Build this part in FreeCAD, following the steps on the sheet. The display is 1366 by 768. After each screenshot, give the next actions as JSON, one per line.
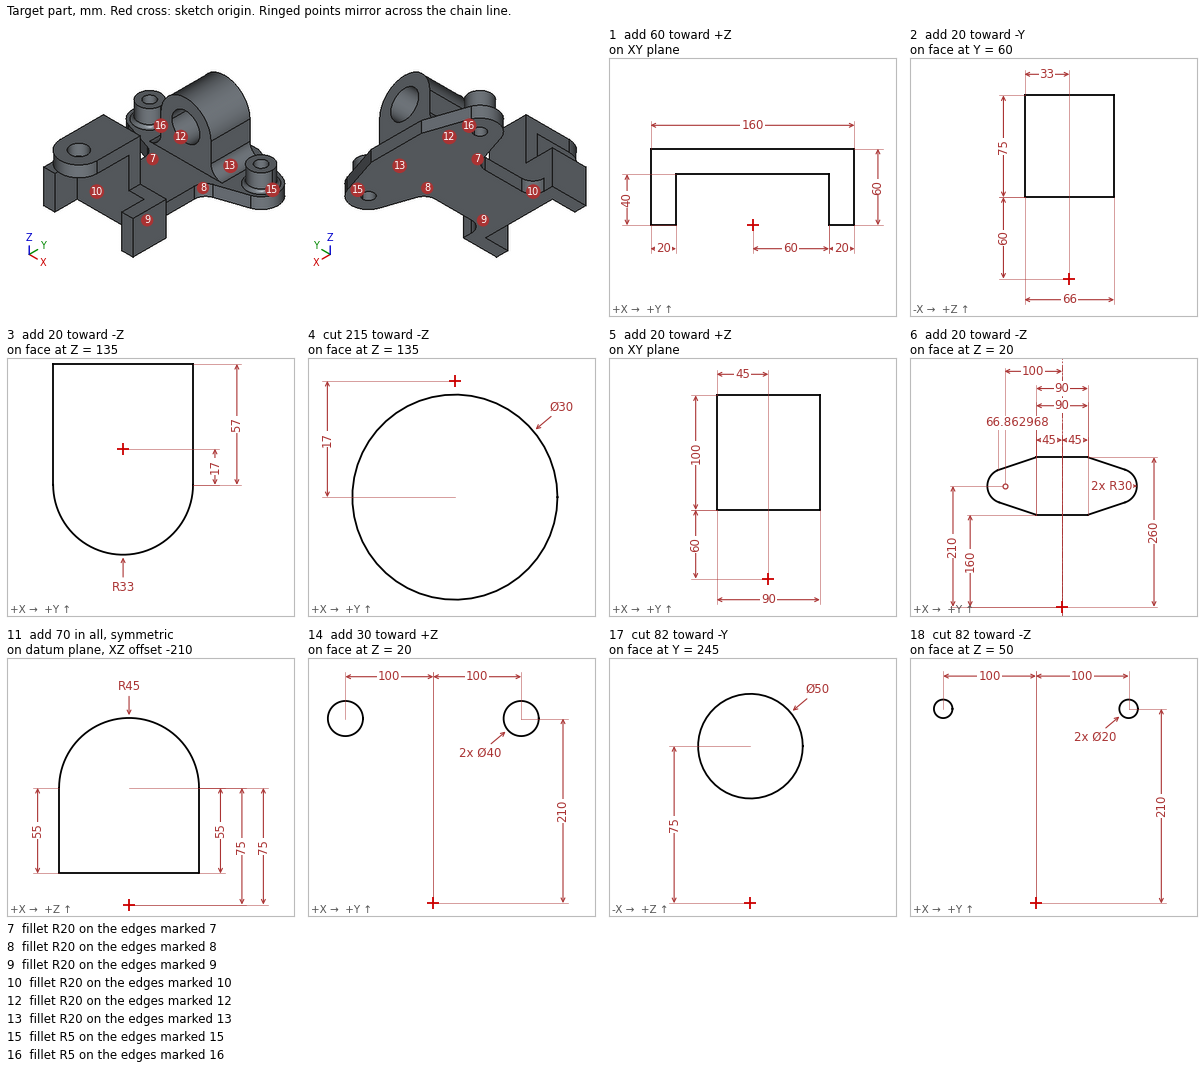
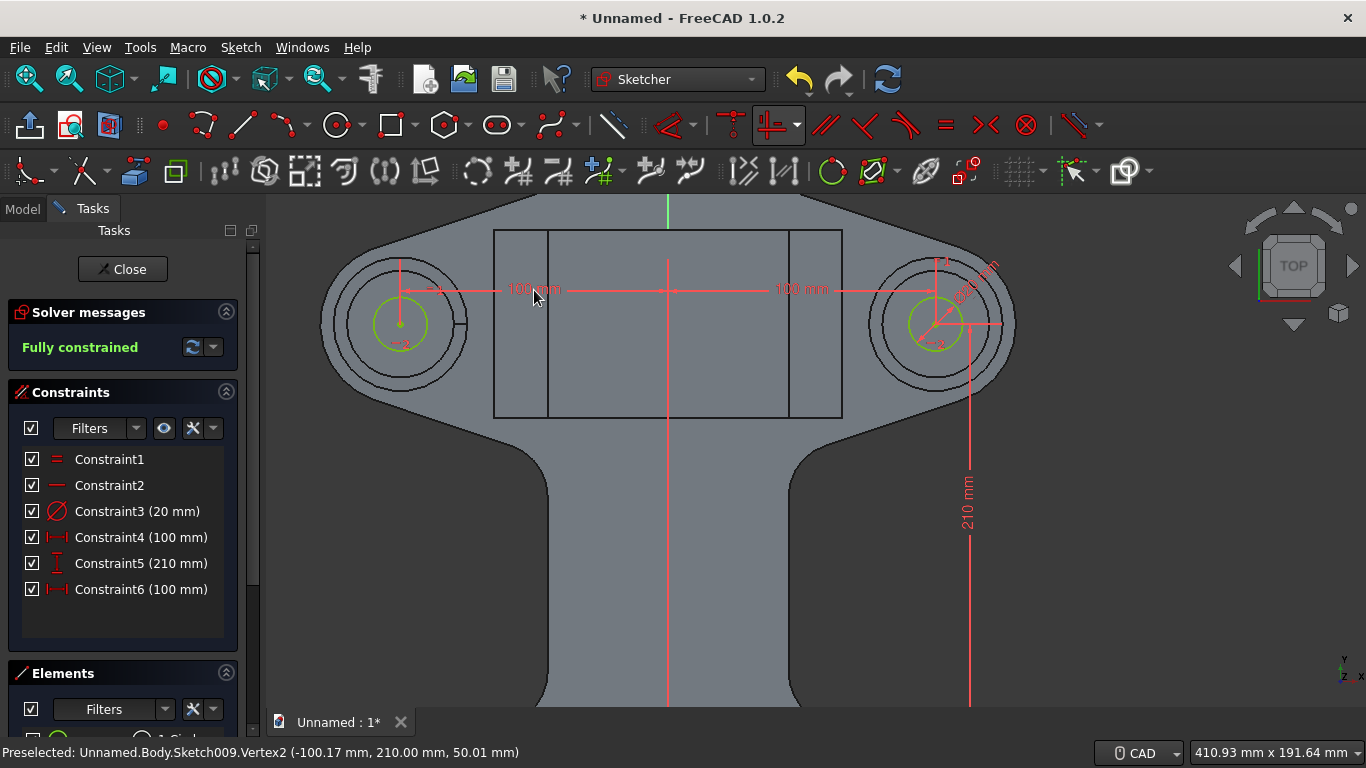
{"action": "left_click", "coordinate": [123, 269]}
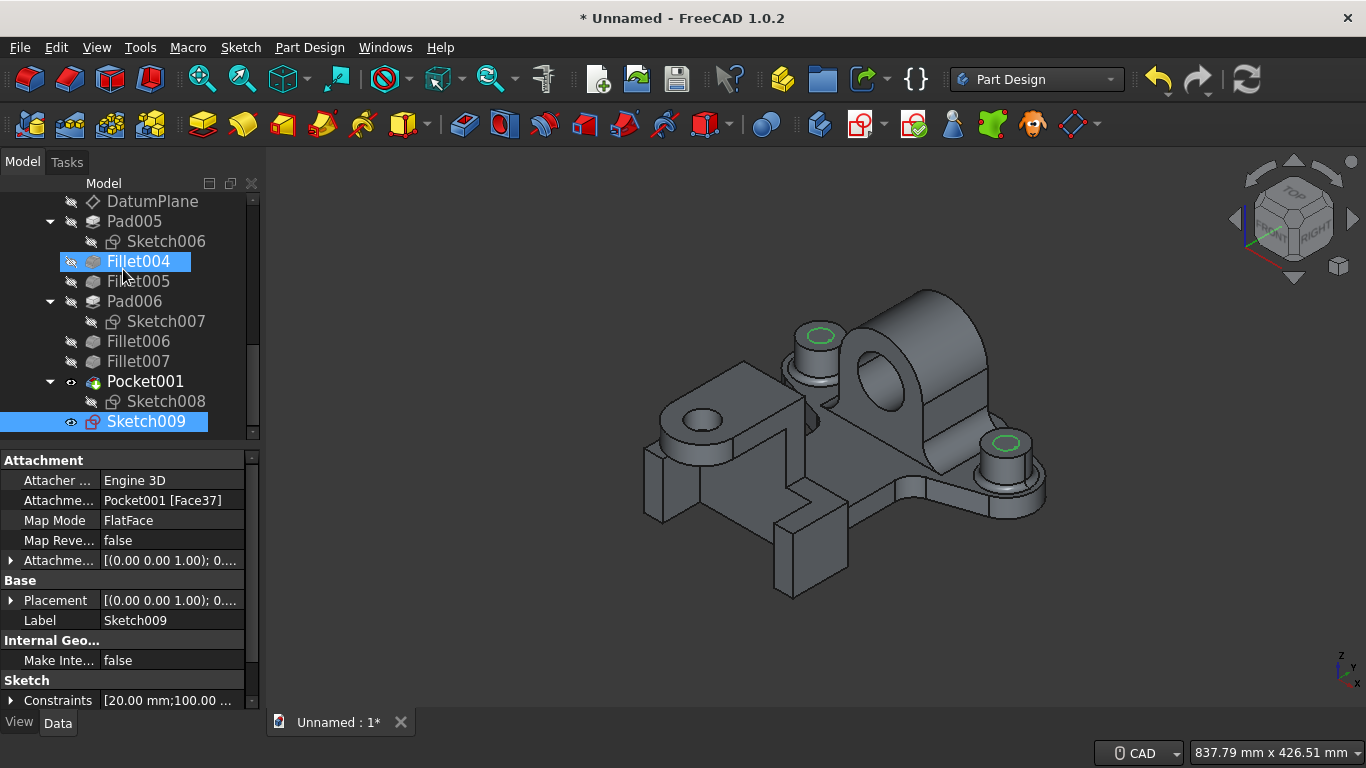
{"action": "left_click", "coordinate": [466, 124]}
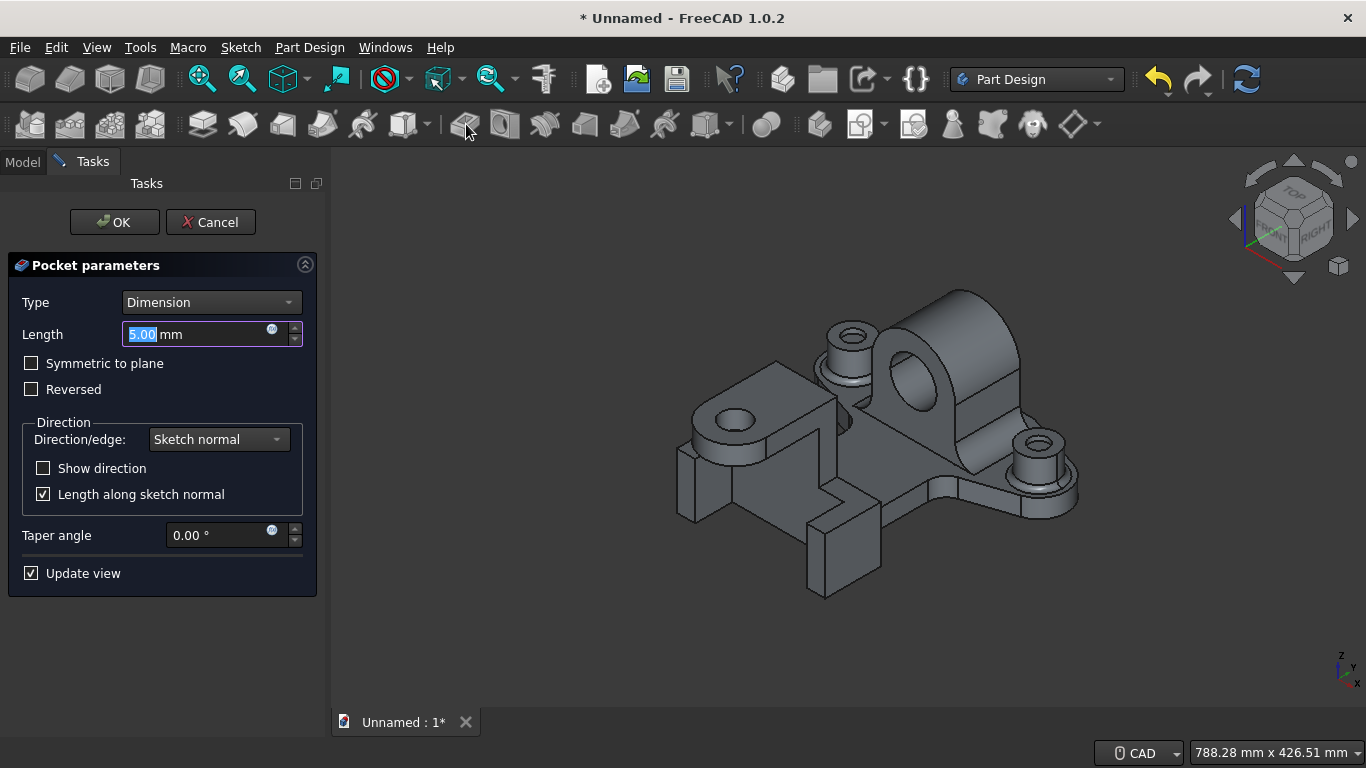
{"action": "type", "text": "82"}
{"action": "key", "text": "Tab"}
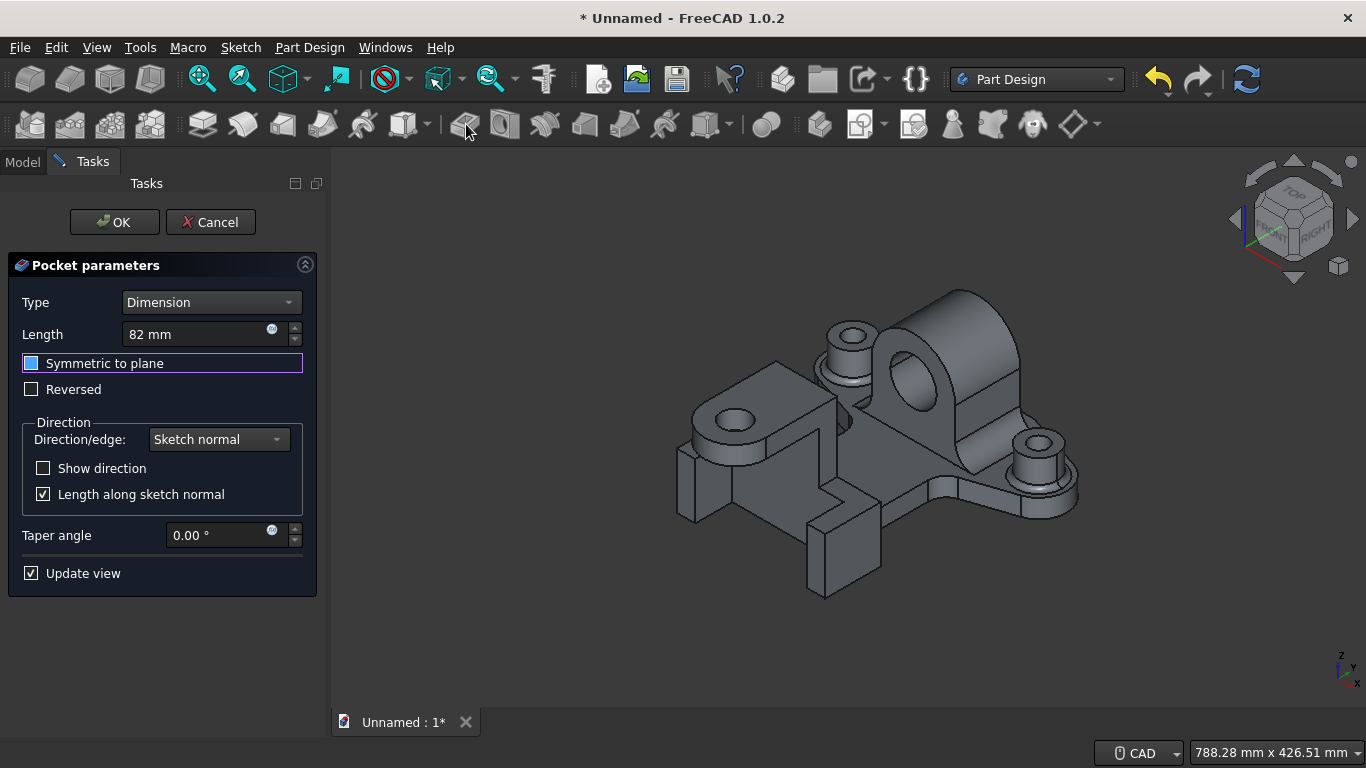
{"action": "left_click", "coordinate": [115, 222]}